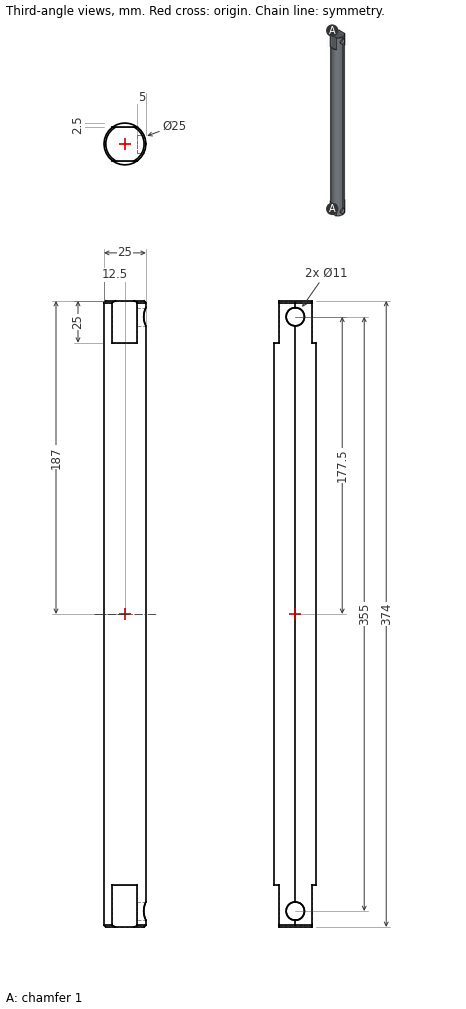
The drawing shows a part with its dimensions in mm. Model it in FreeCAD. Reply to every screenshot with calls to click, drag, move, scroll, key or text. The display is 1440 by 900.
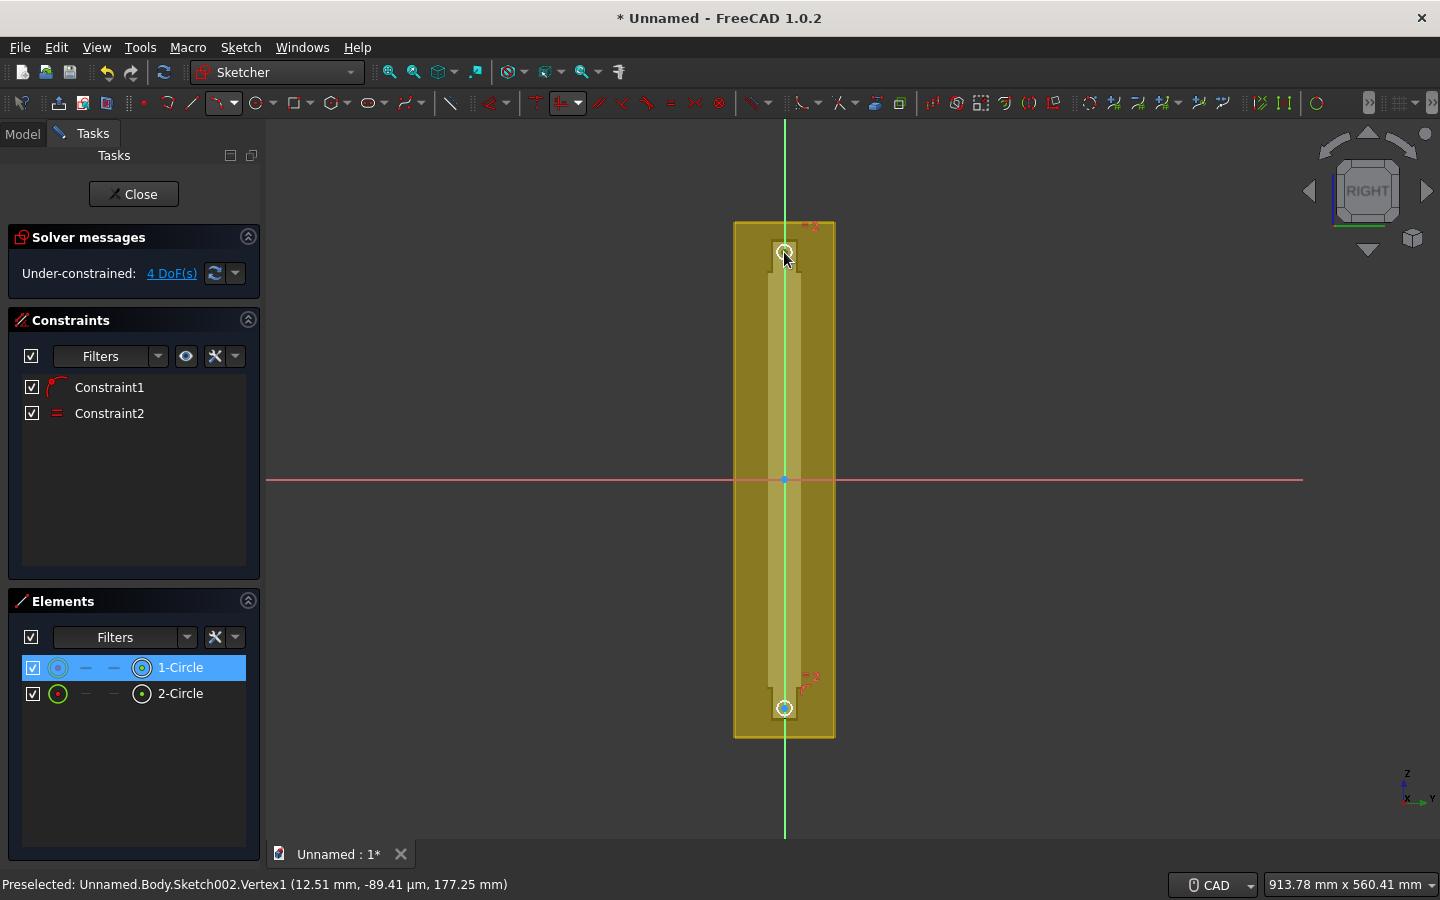
click(785, 764)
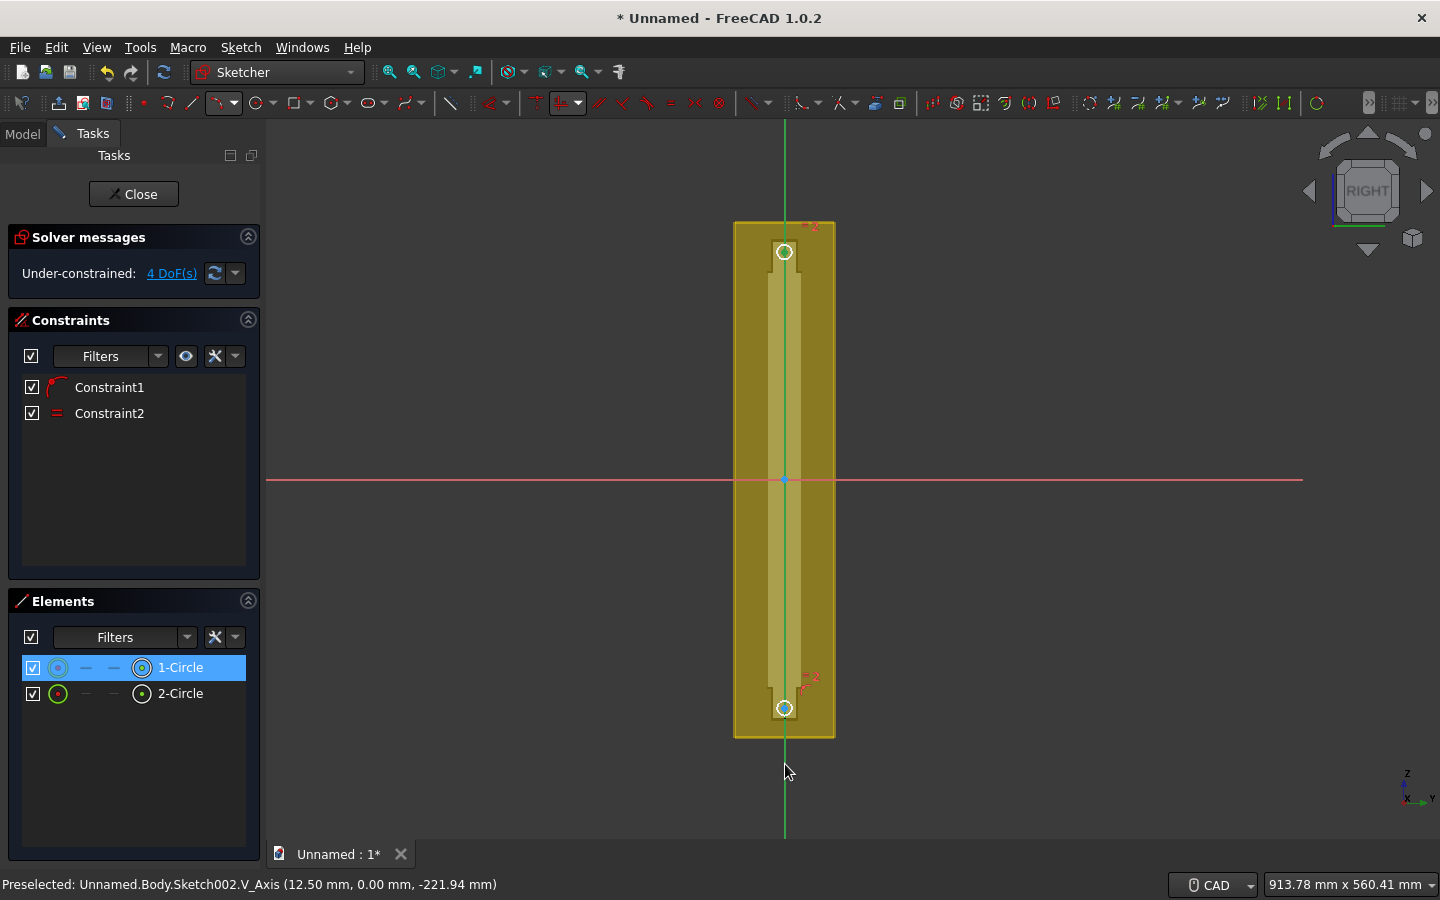
click(536, 104)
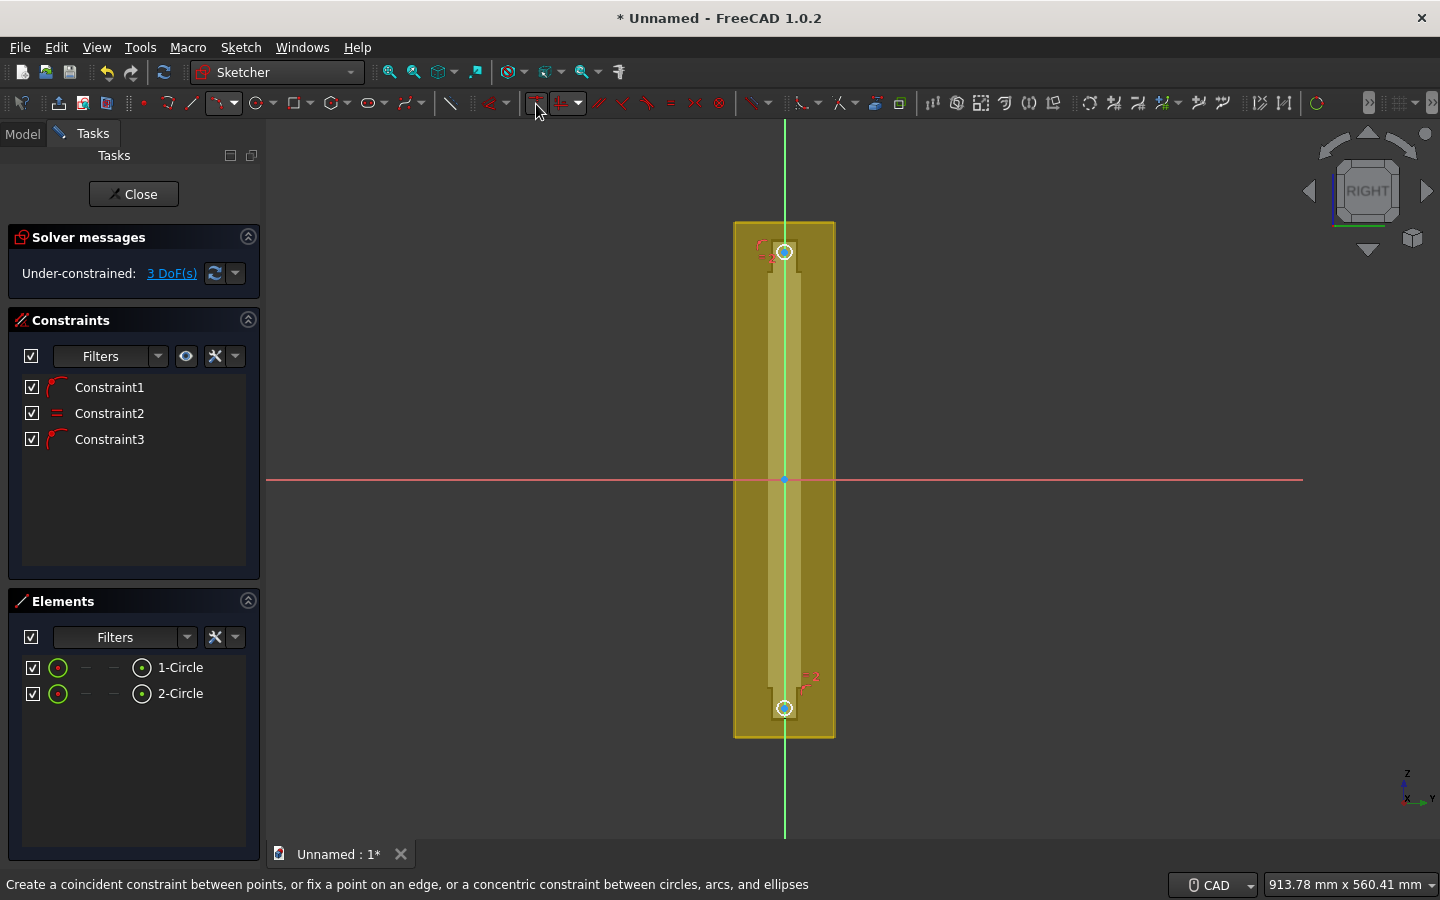
click(490, 104)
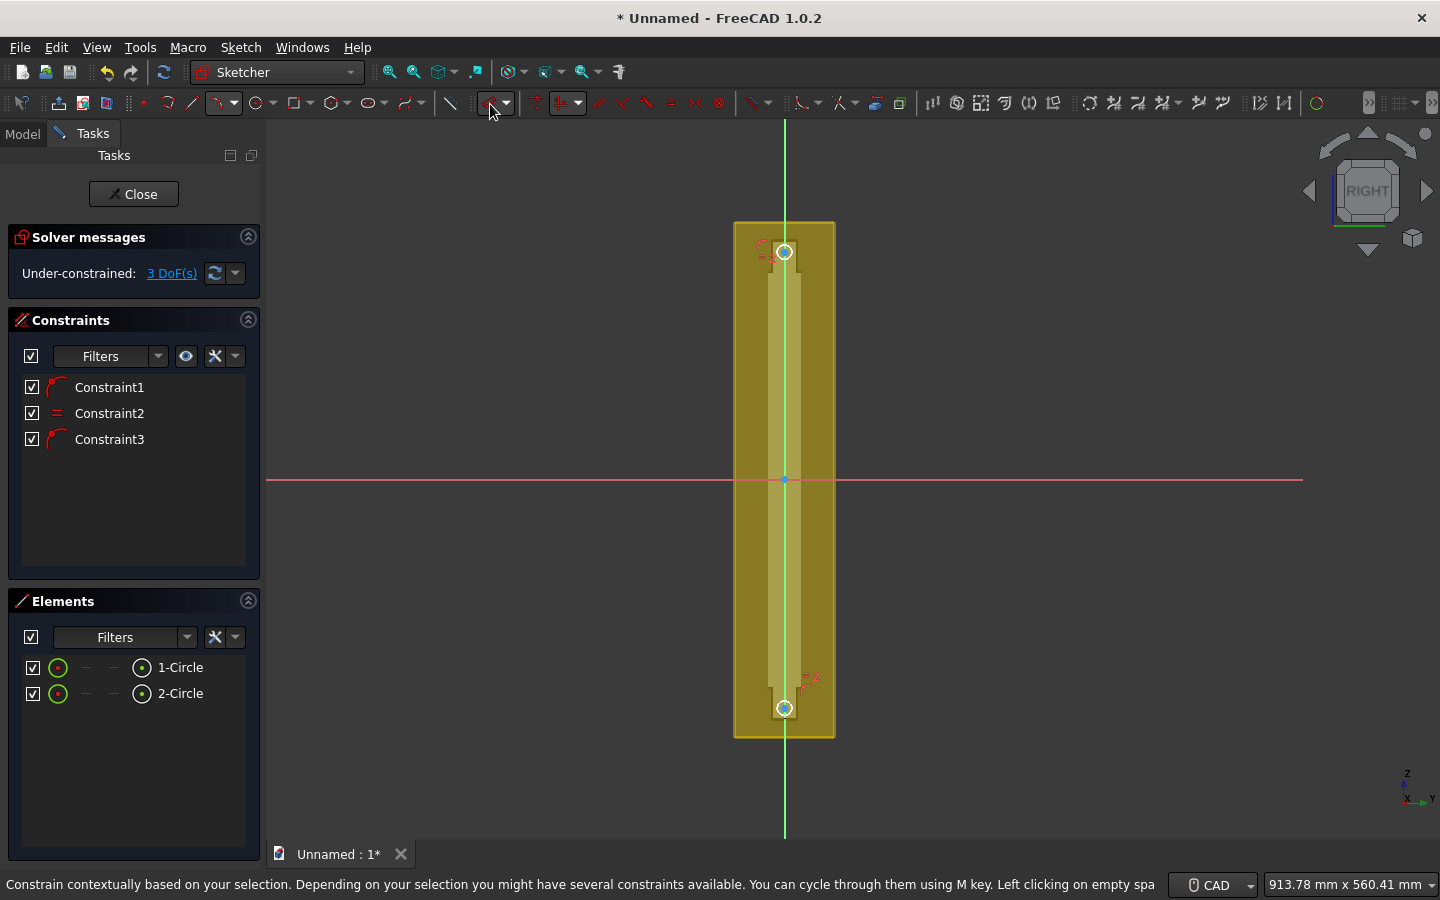
scroll(785, 245, up, 6)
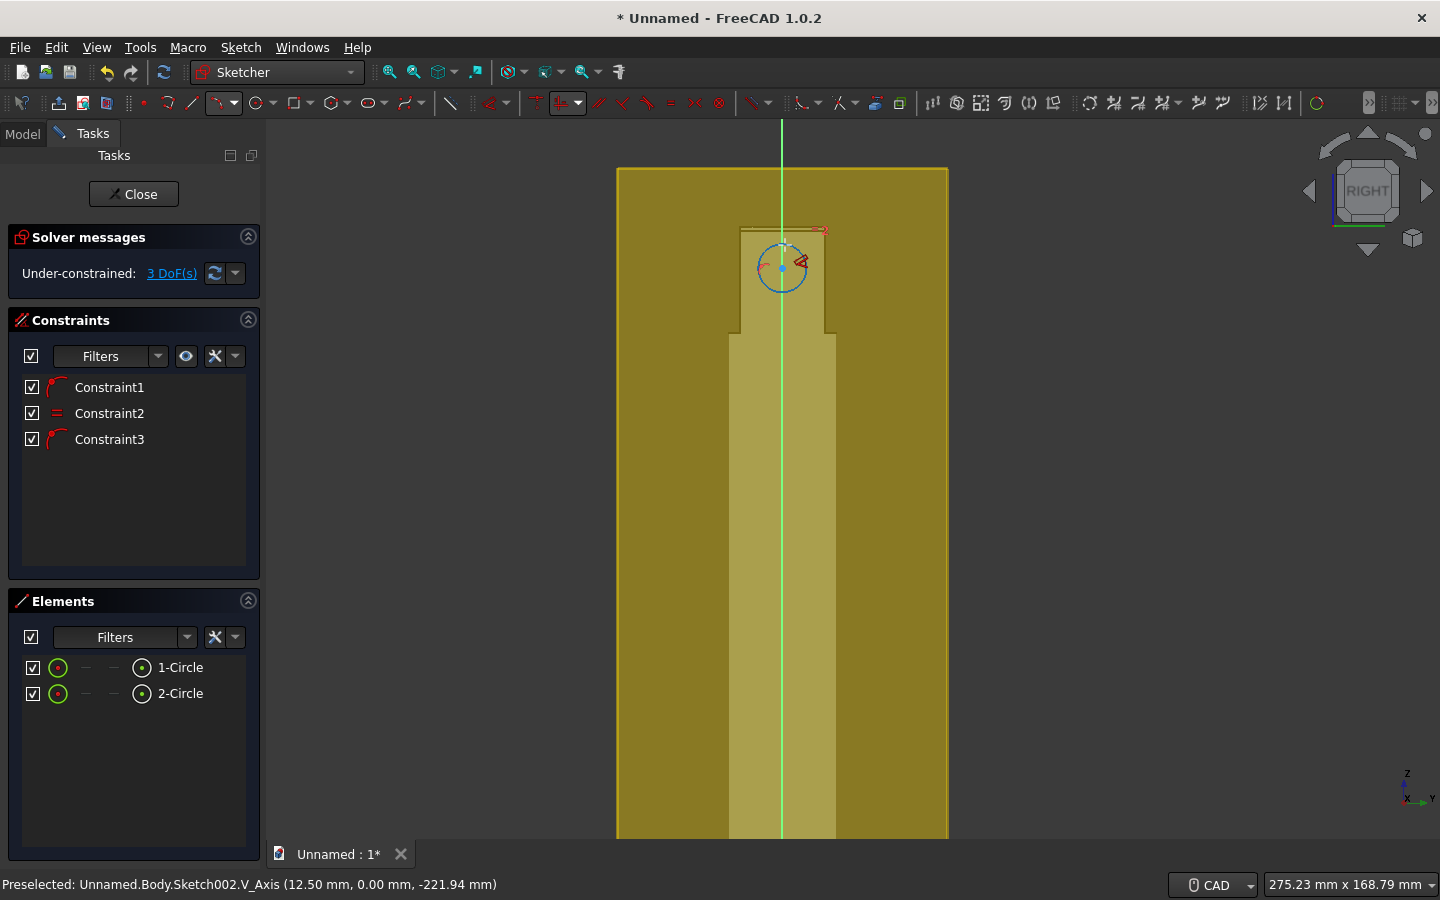
click(783, 244)
click(811, 220)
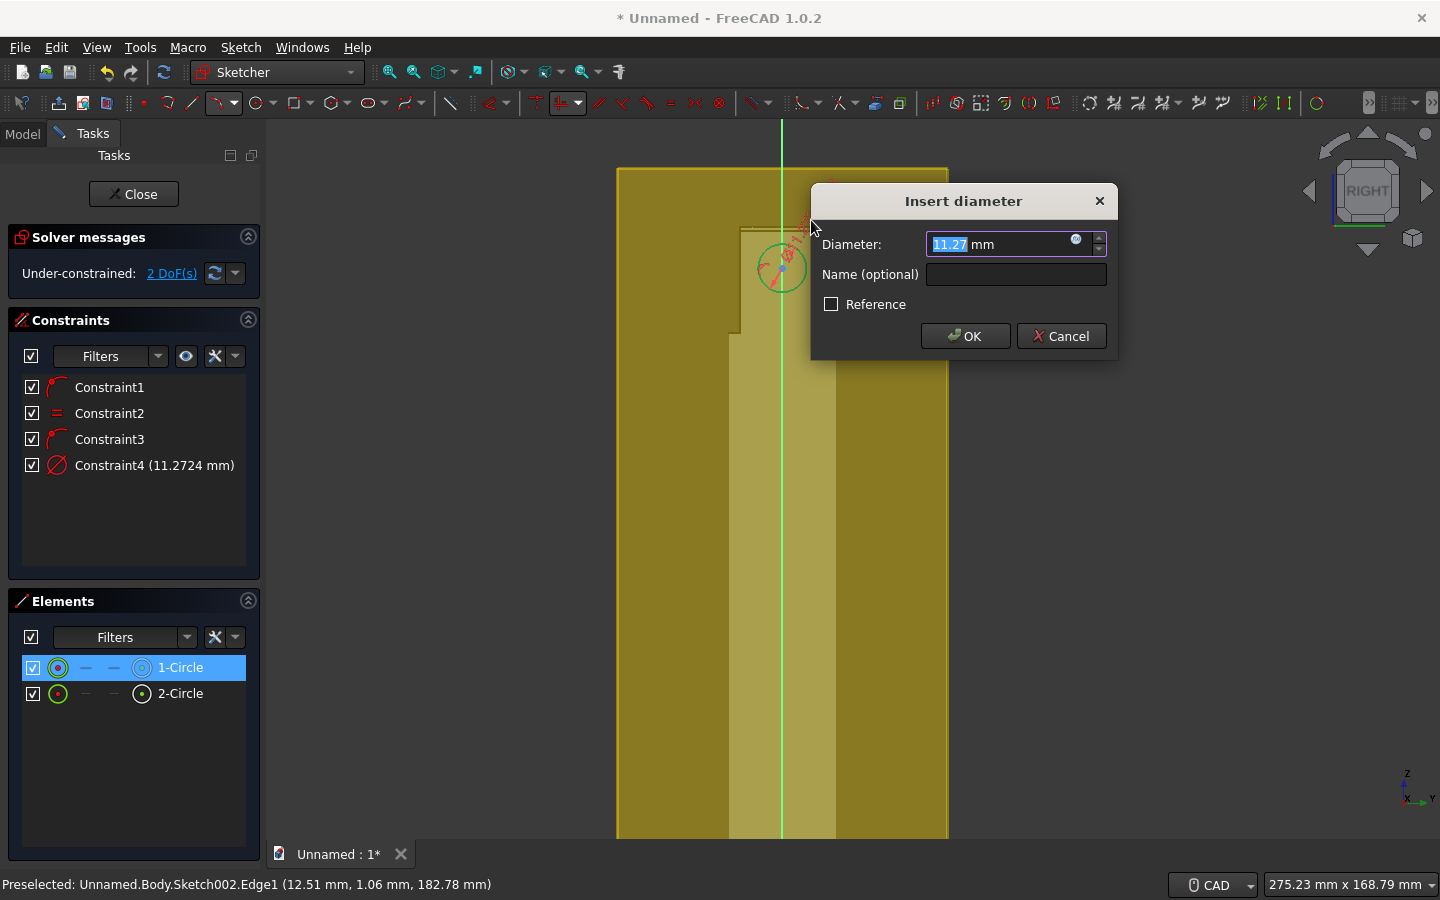
text(11)
key(Return)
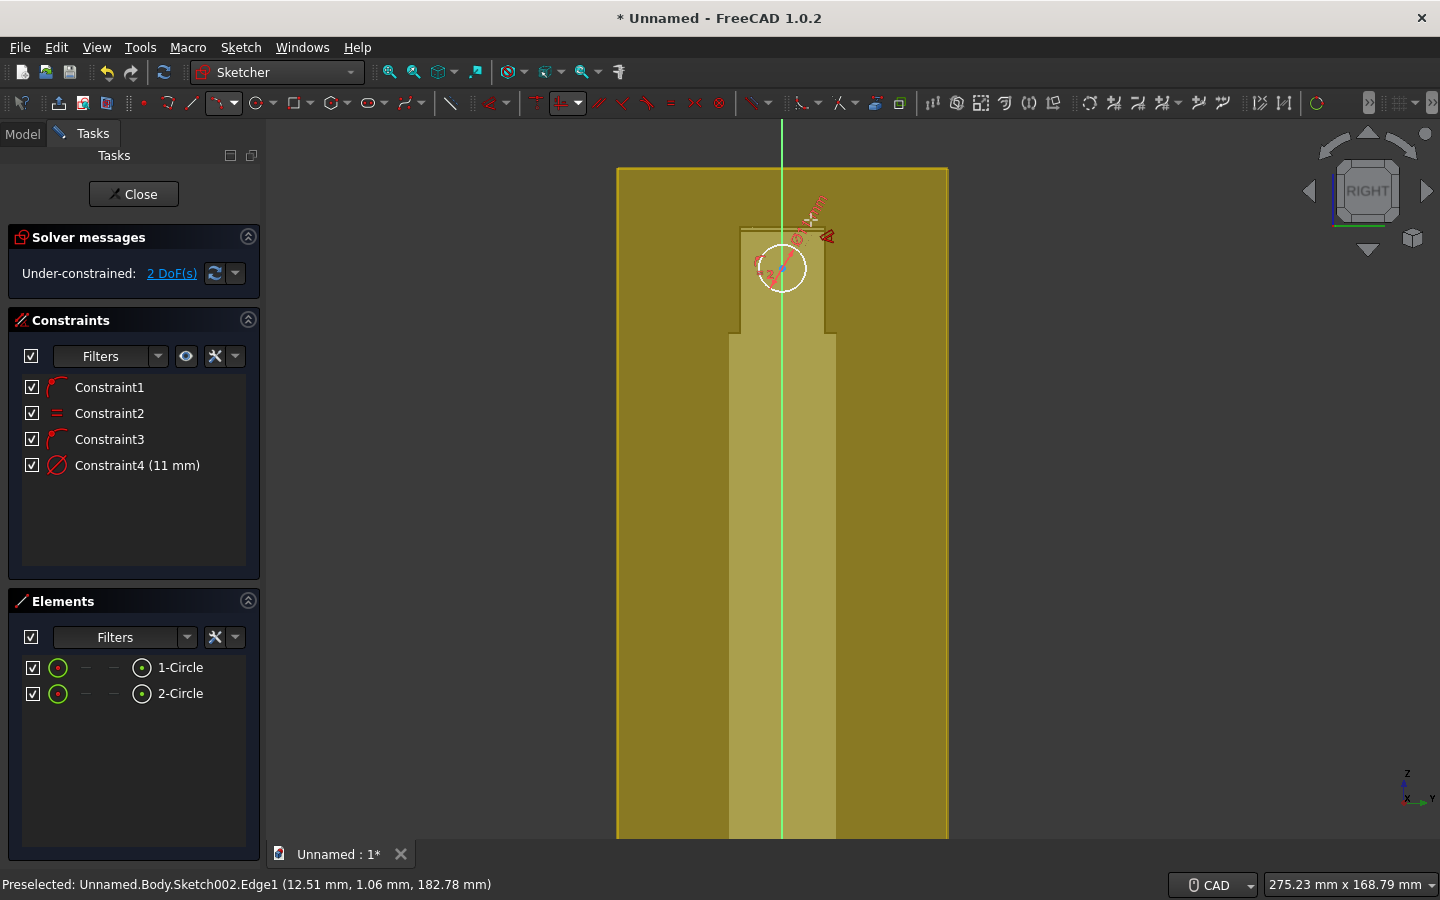
click(782, 268)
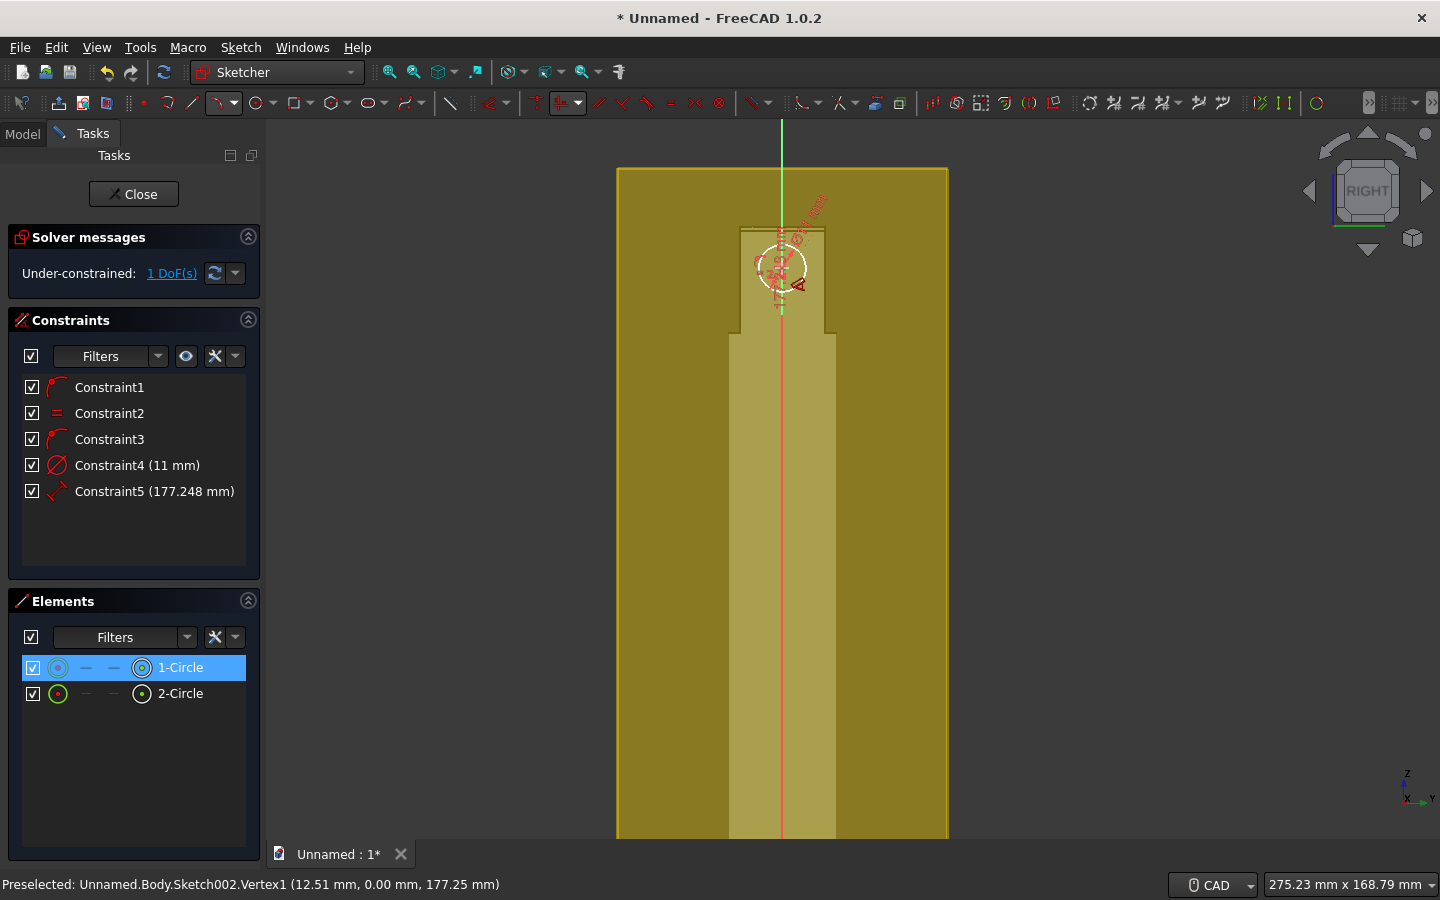
scroll(785, 244, down, 6)